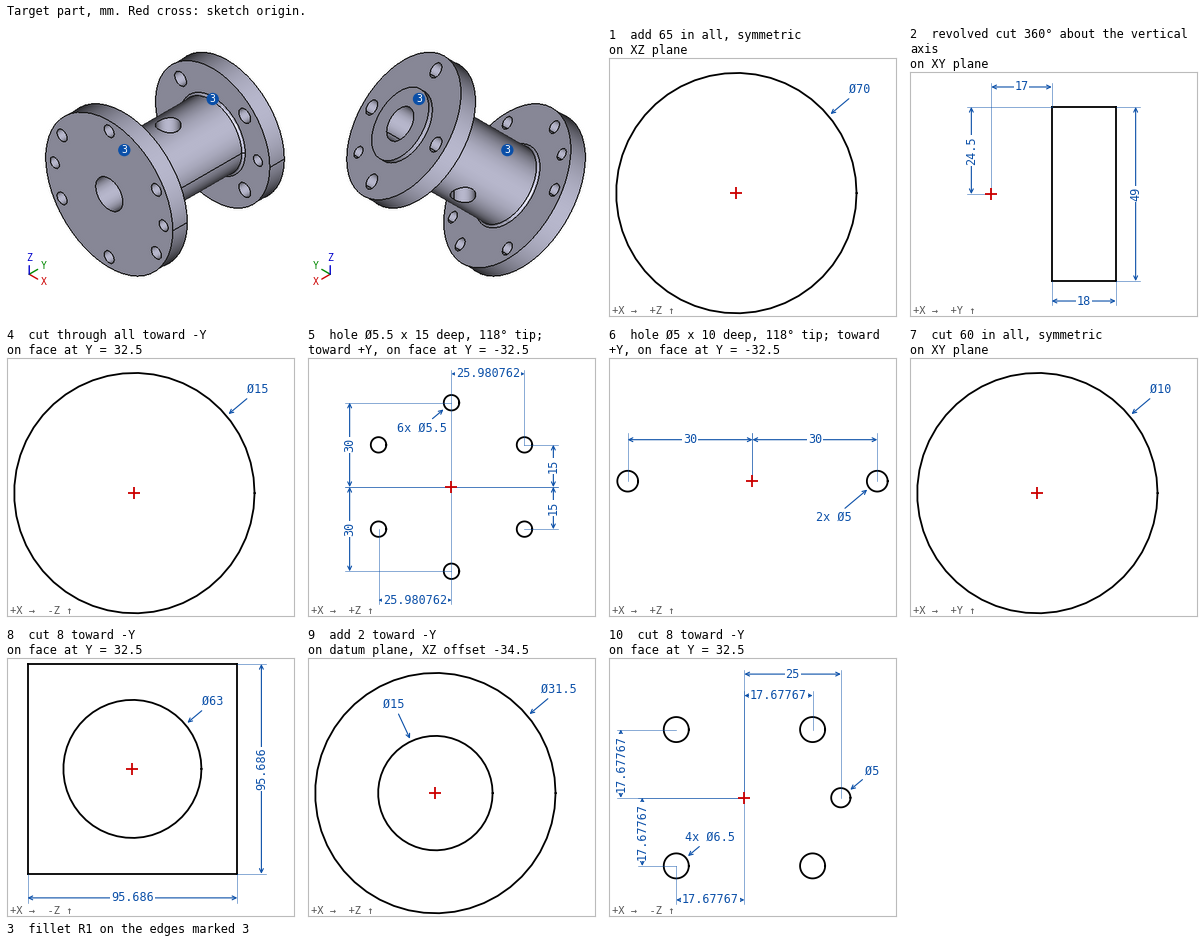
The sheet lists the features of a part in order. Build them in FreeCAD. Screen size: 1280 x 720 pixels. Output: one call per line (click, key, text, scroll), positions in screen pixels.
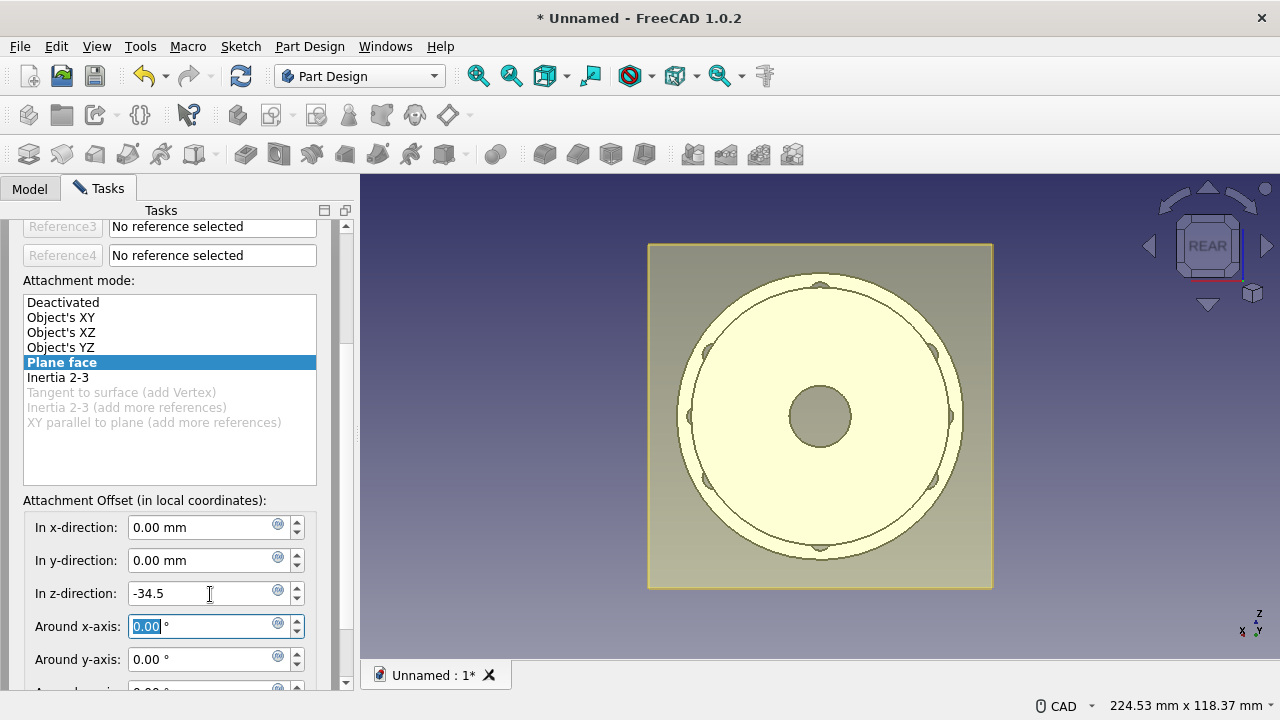
scroll(346, 455, up, 4)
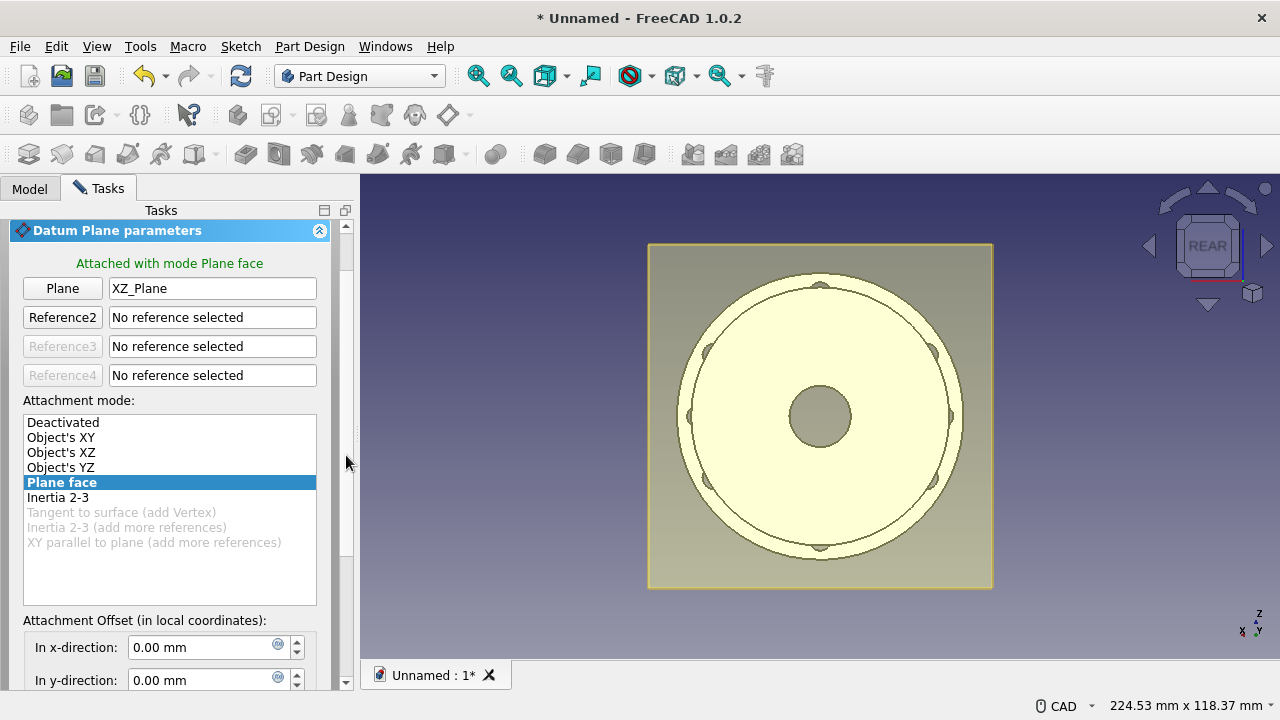
click(127, 249)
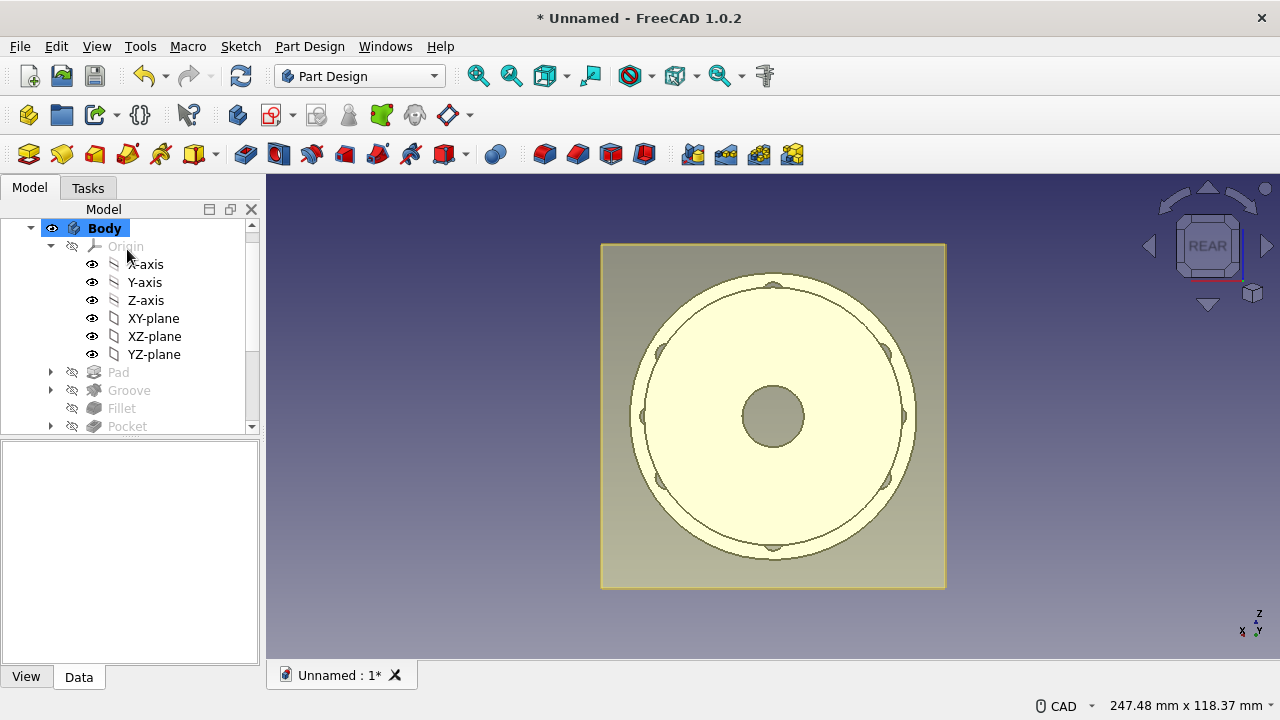
scroll(121, 332, down, 3)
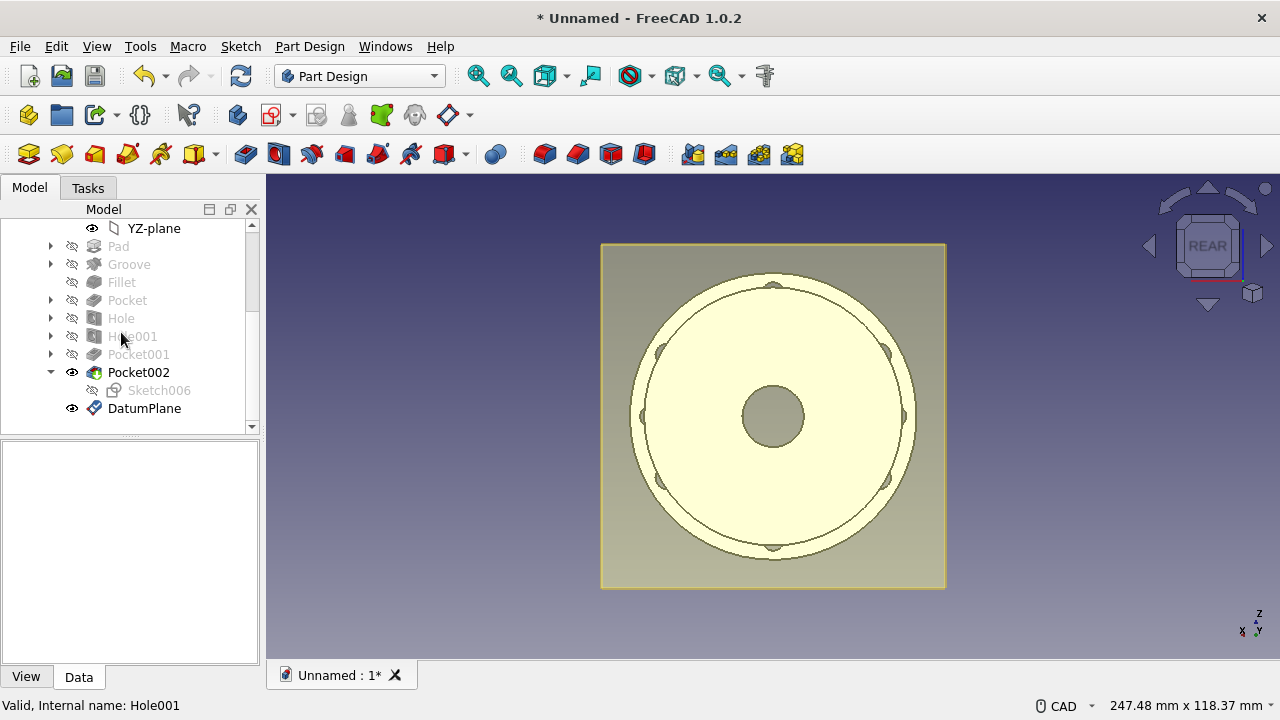
click(117, 408)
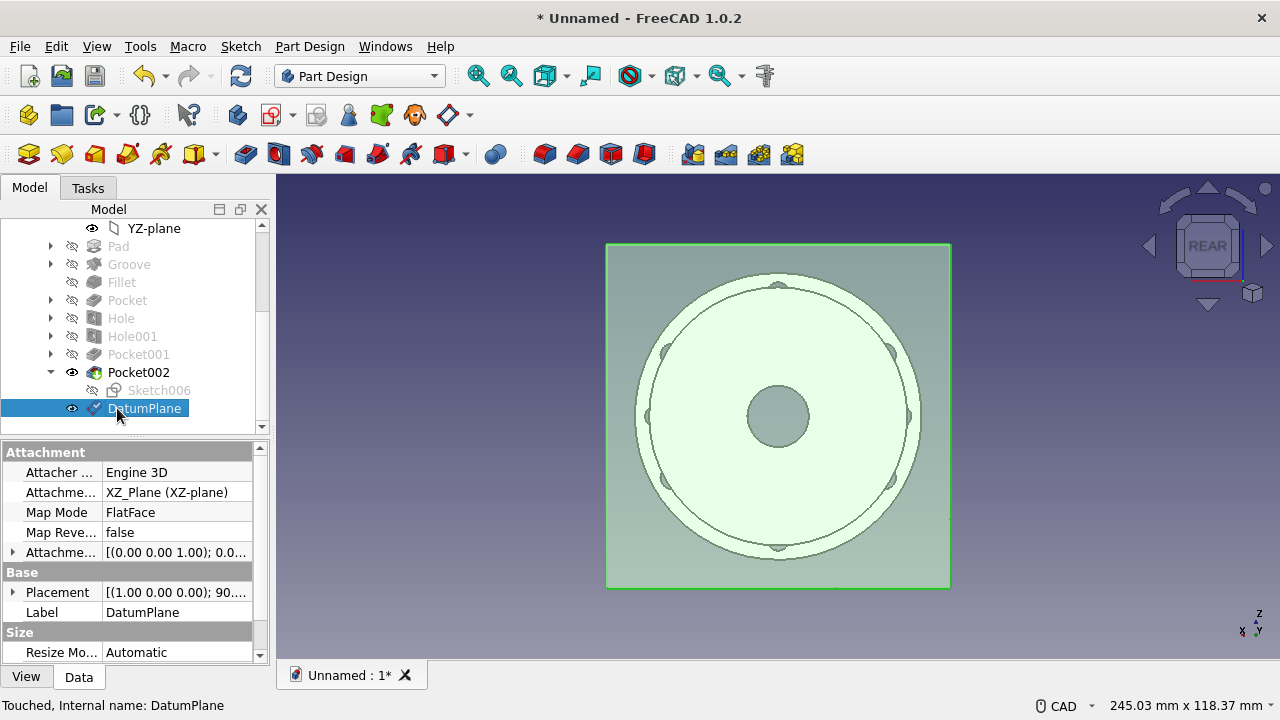
click(270, 116)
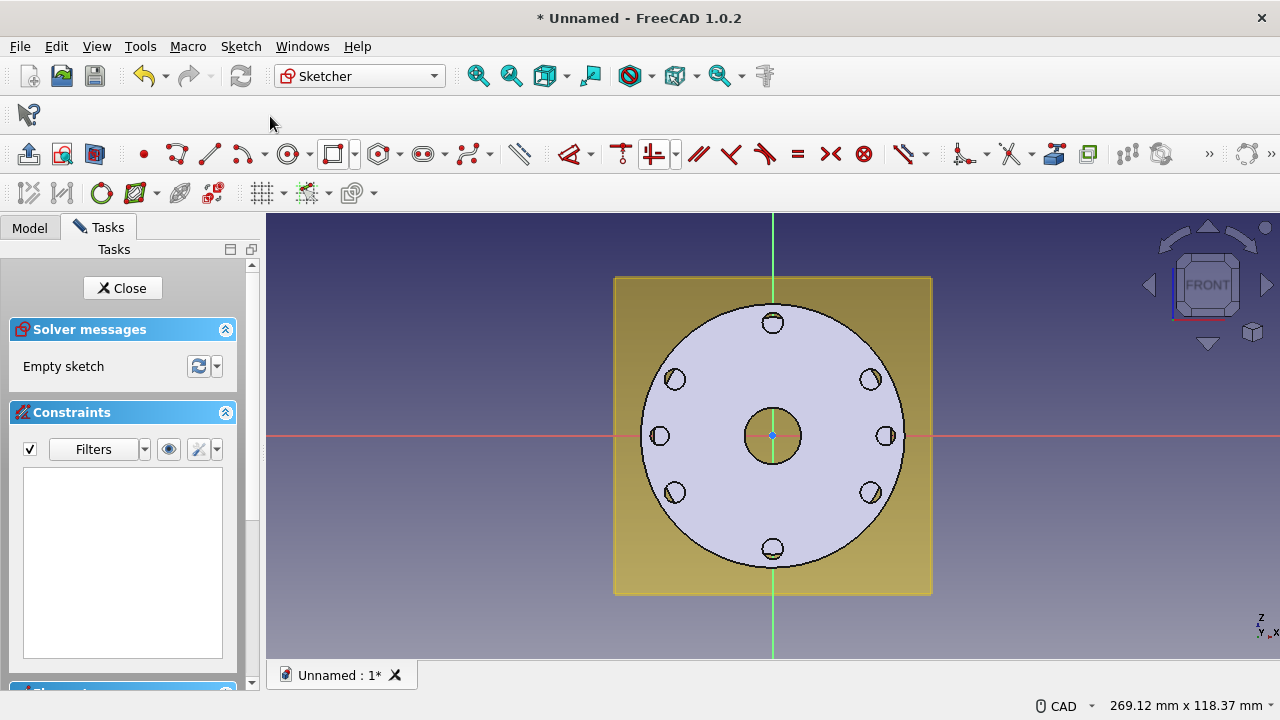
click(95, 154)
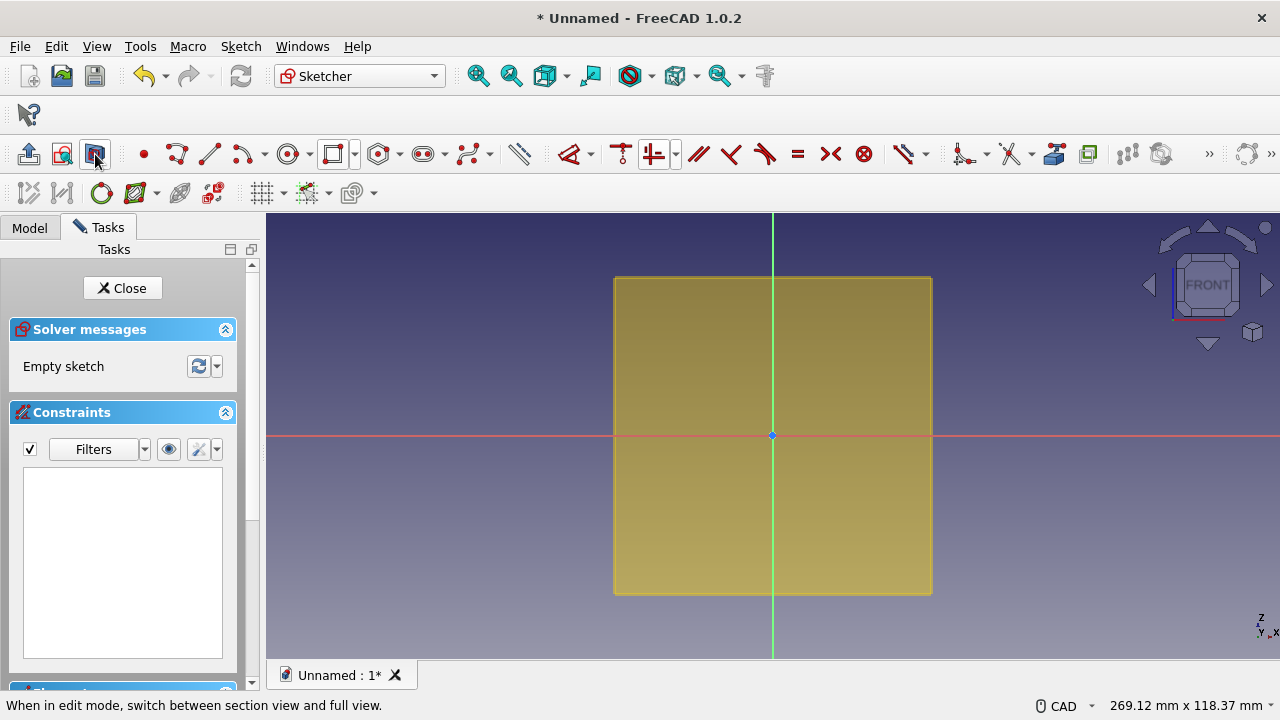
scroll(829, 436, up, 4)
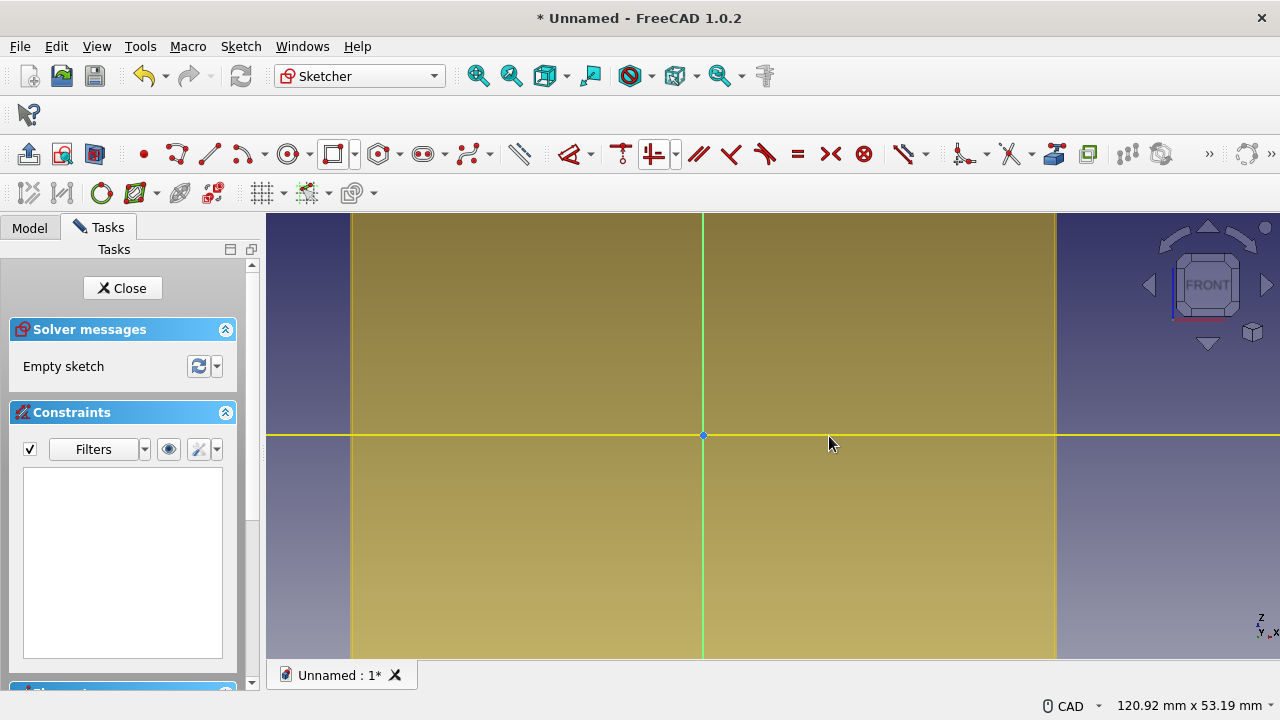
click(288, 154)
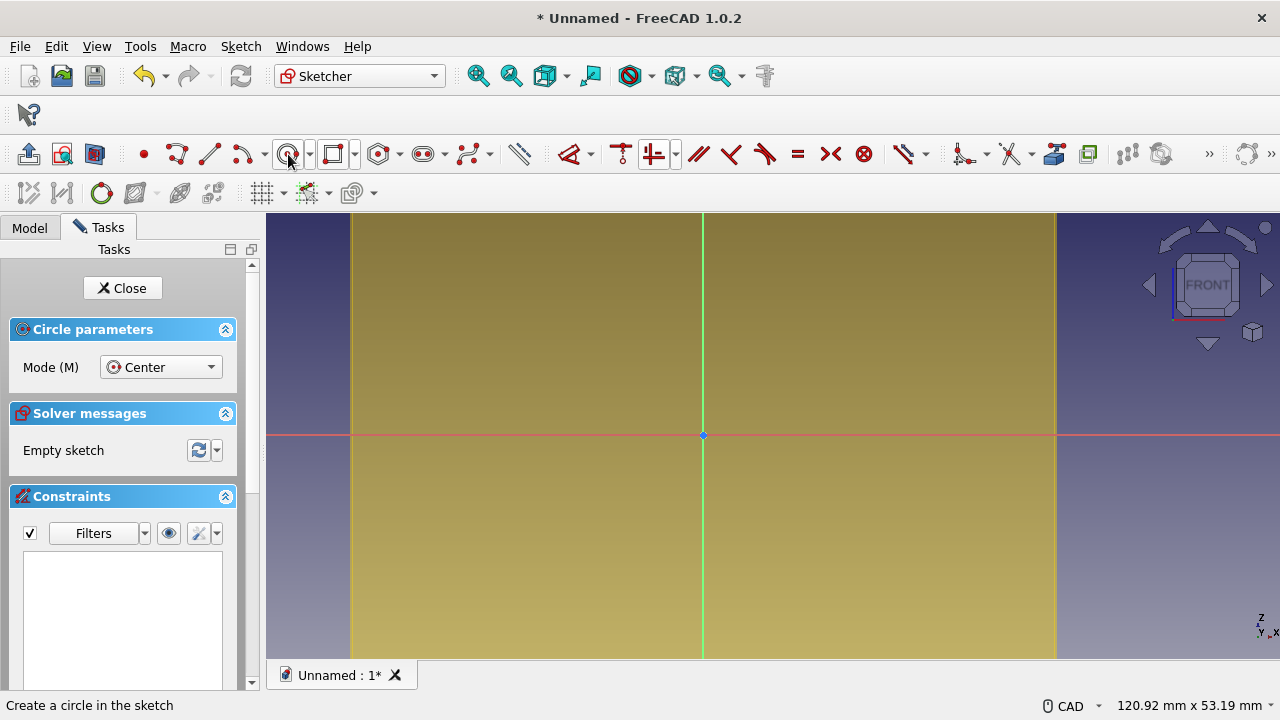
click(703, 435)
move(797, 342)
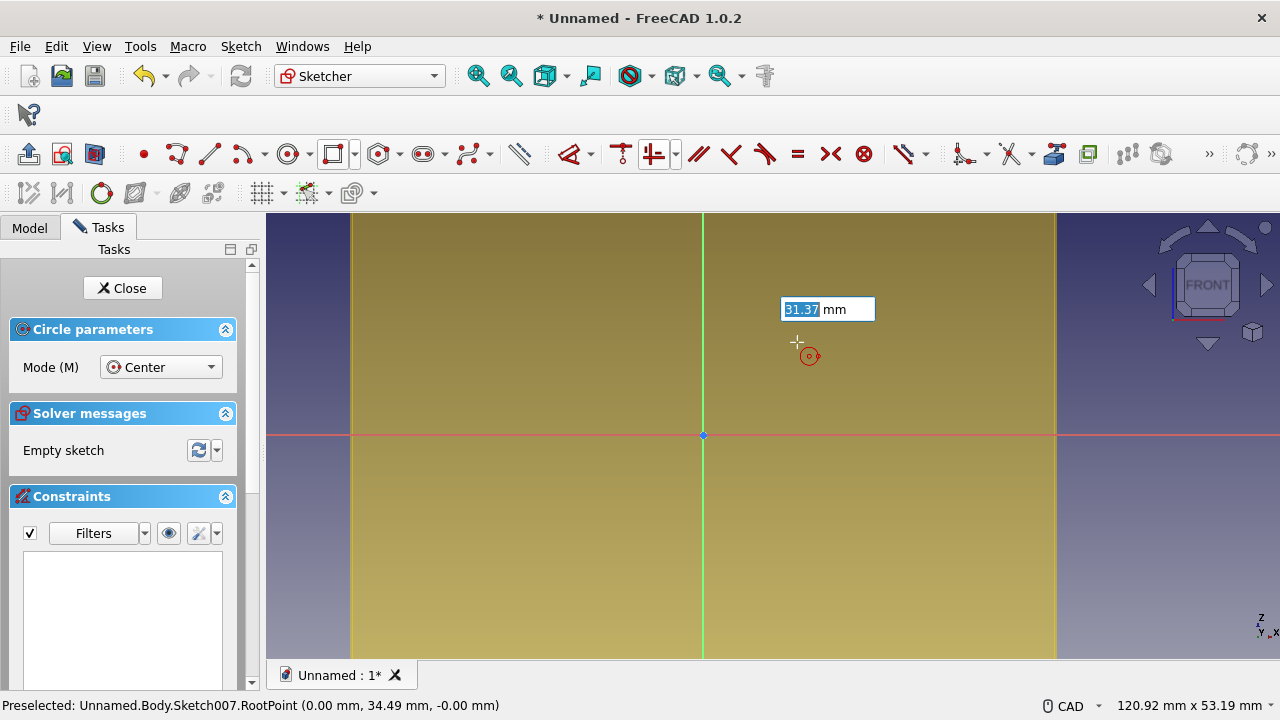
text(31.5)
key(Return)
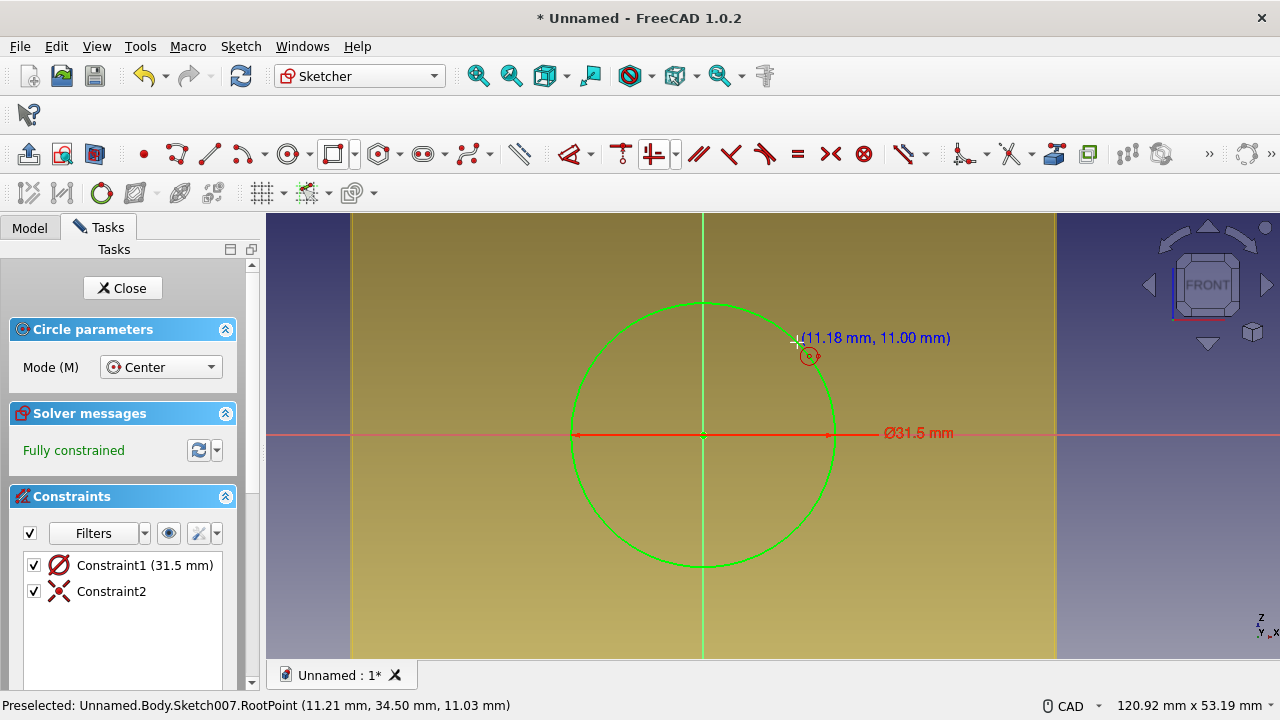
click(703, 435)
move(748, 391)